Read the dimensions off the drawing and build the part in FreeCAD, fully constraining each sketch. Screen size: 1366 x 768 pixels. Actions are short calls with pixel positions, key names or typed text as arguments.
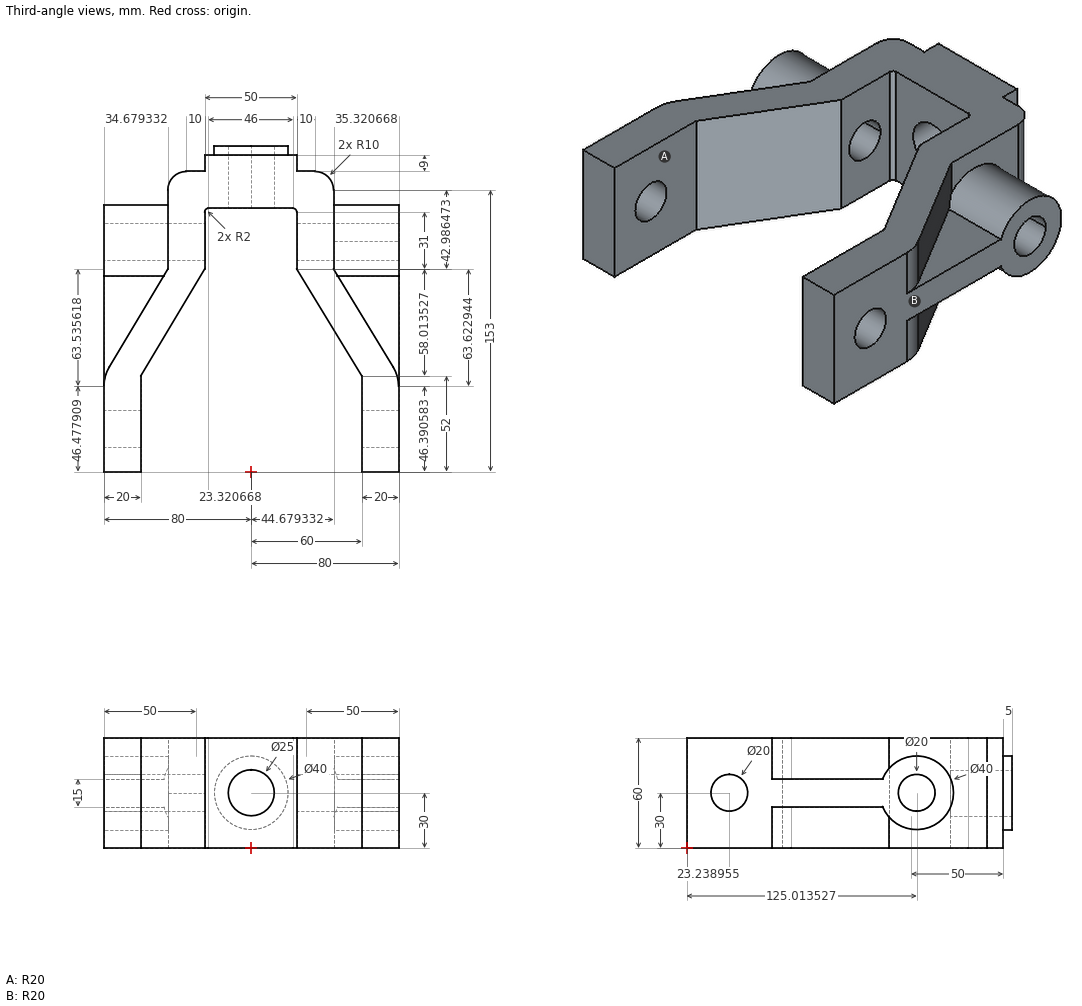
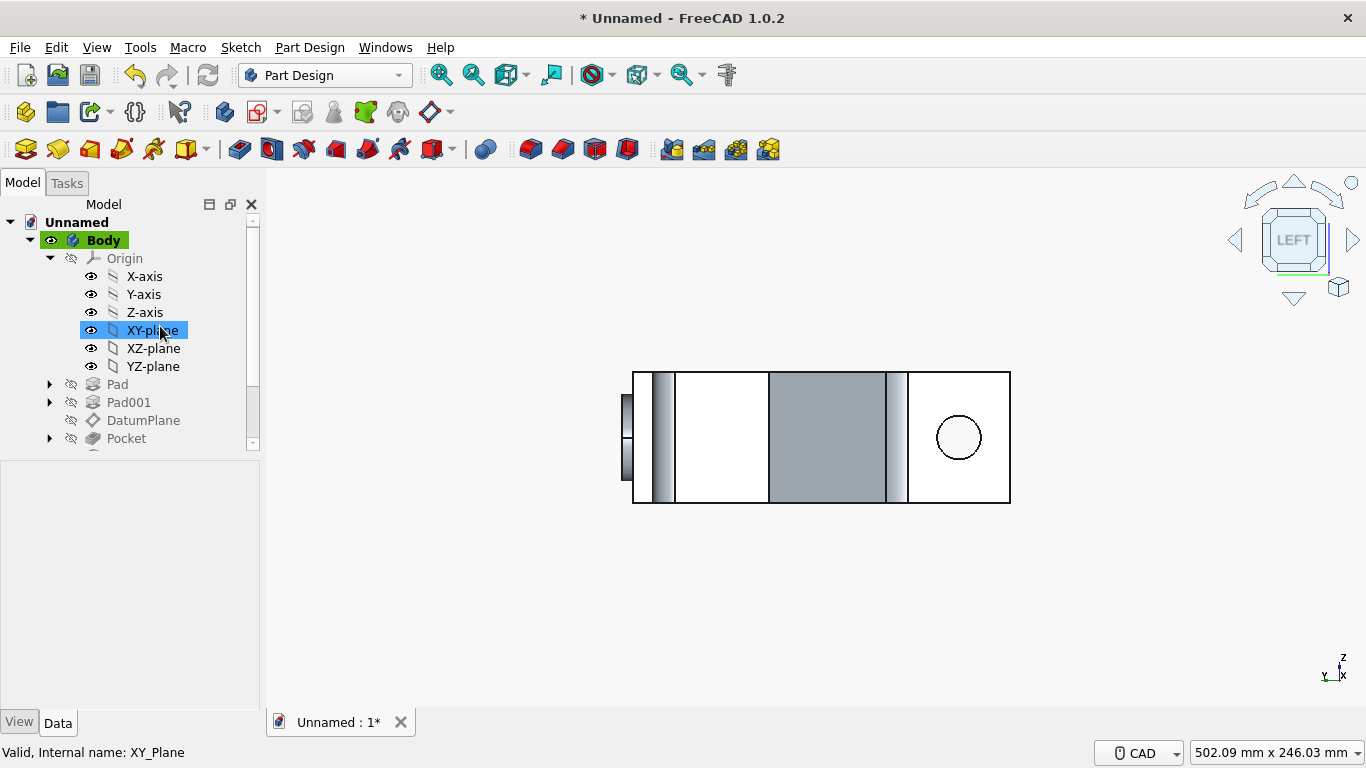
click(136, 366)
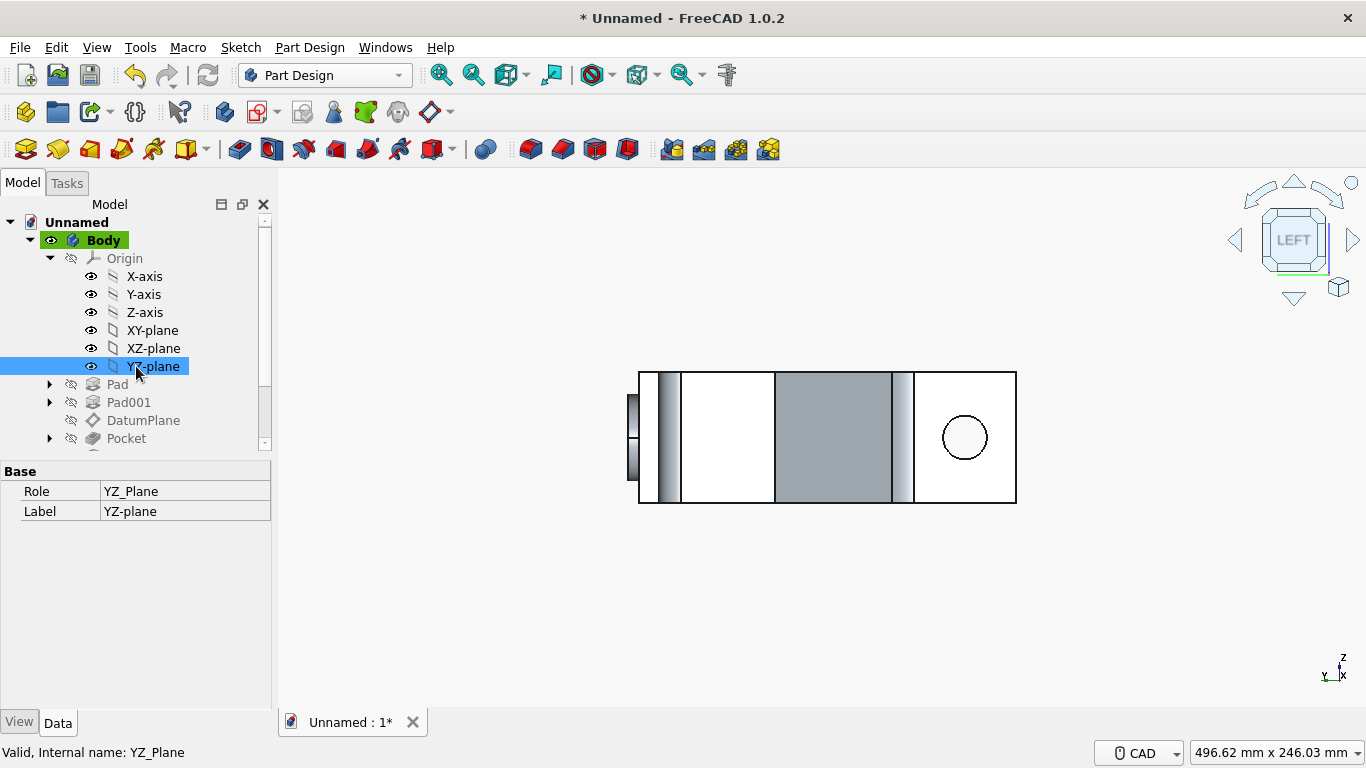
click(430, 112)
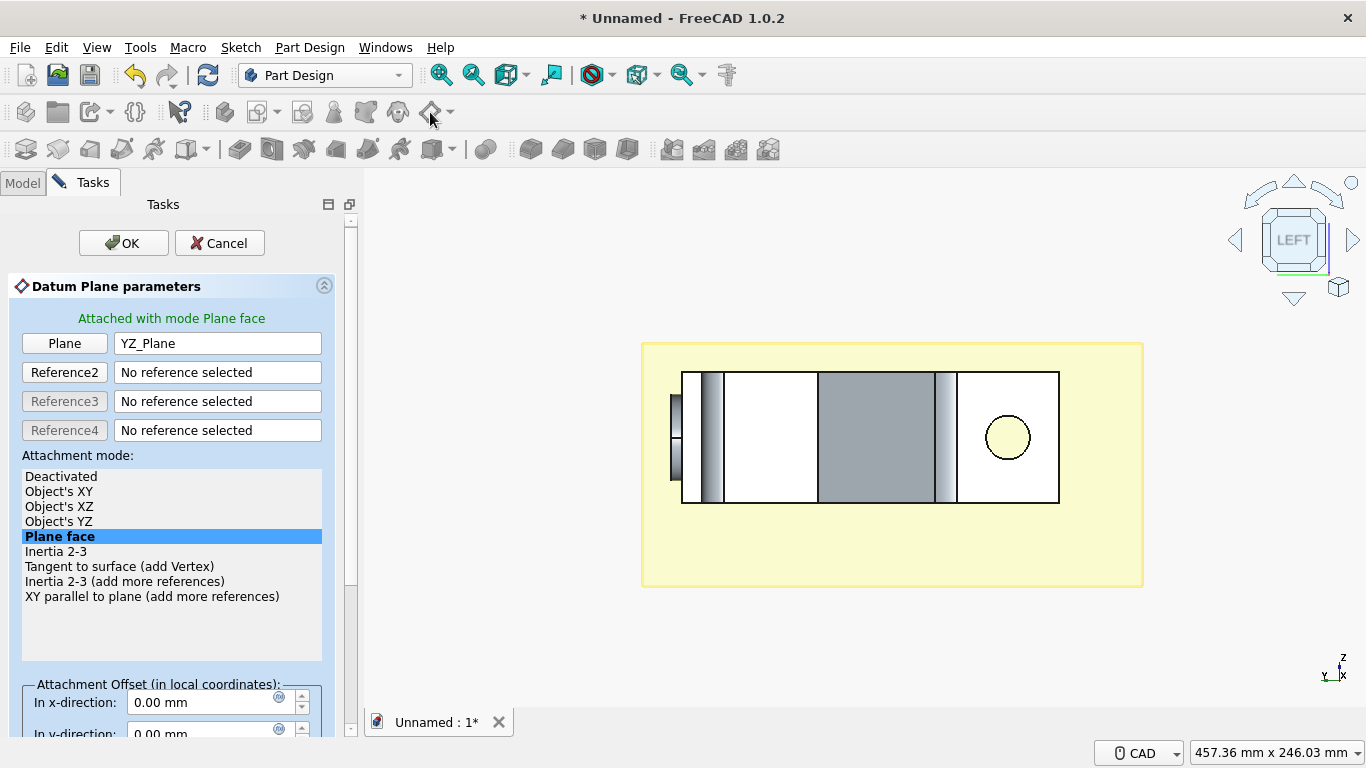
scroll(351, 475, down, 2)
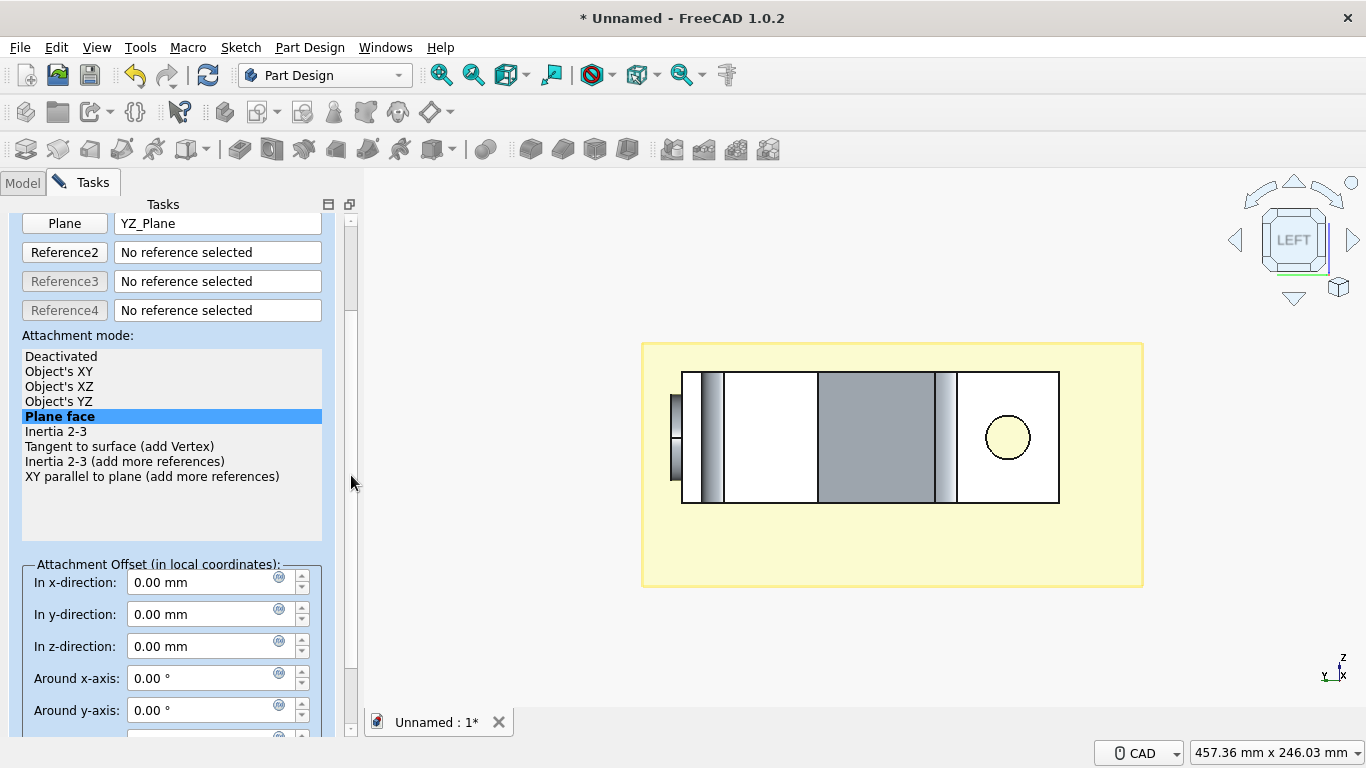
triple_click(210, 646)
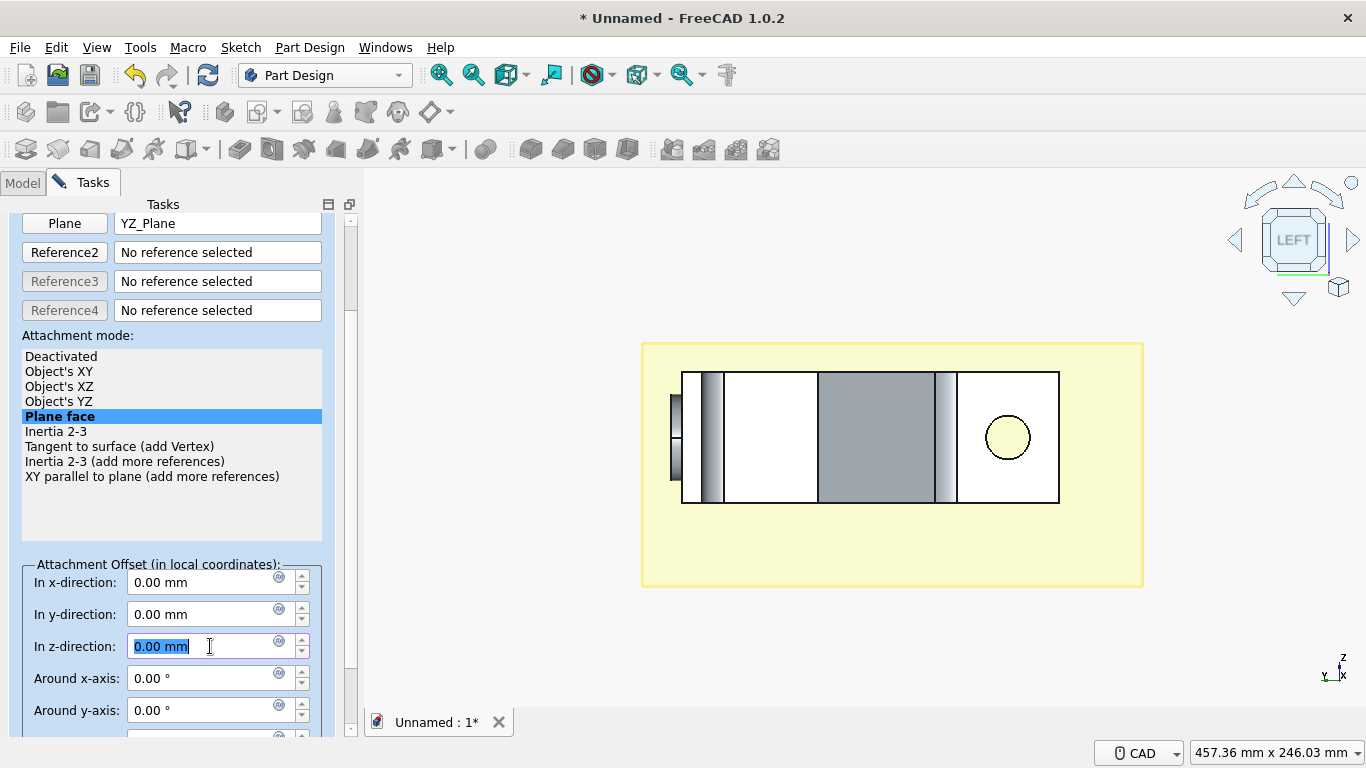
text(30)
key(Tab)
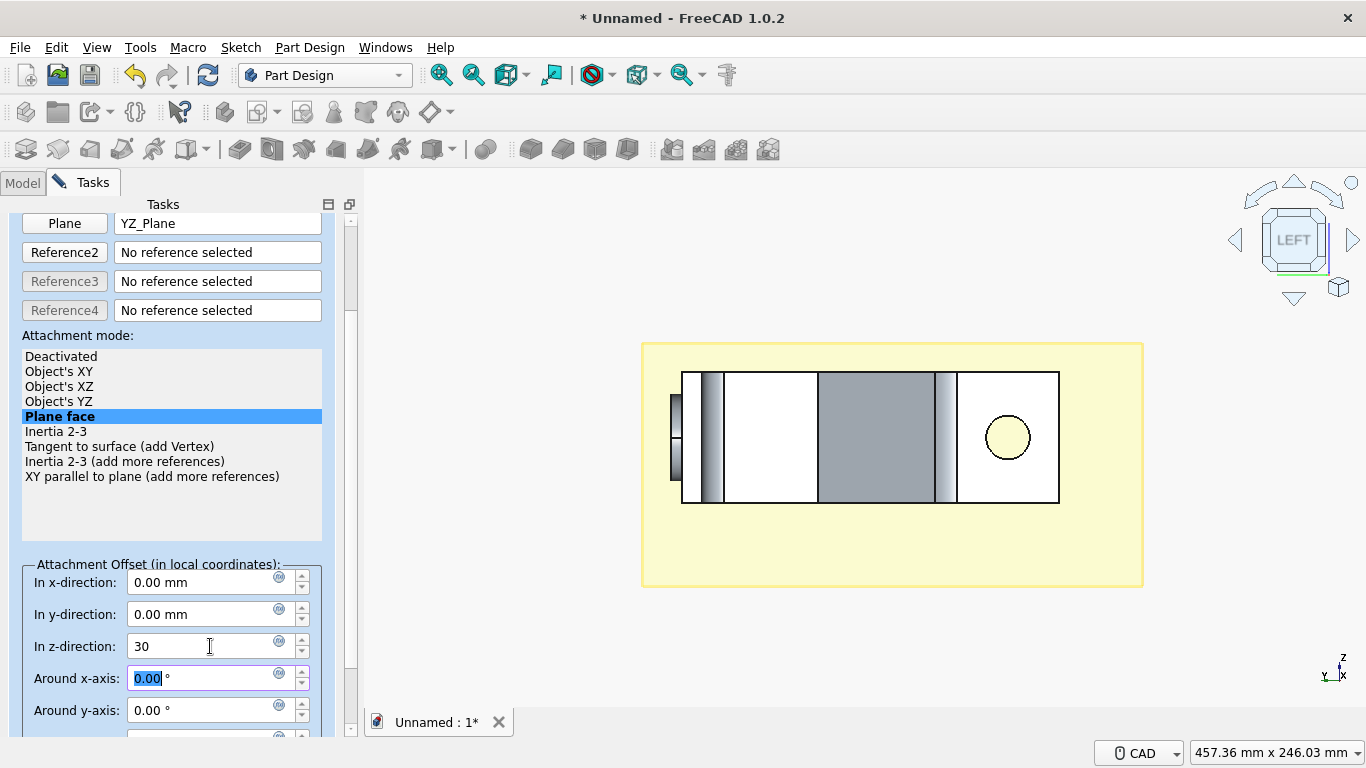
scroll(351, 475, up, 3)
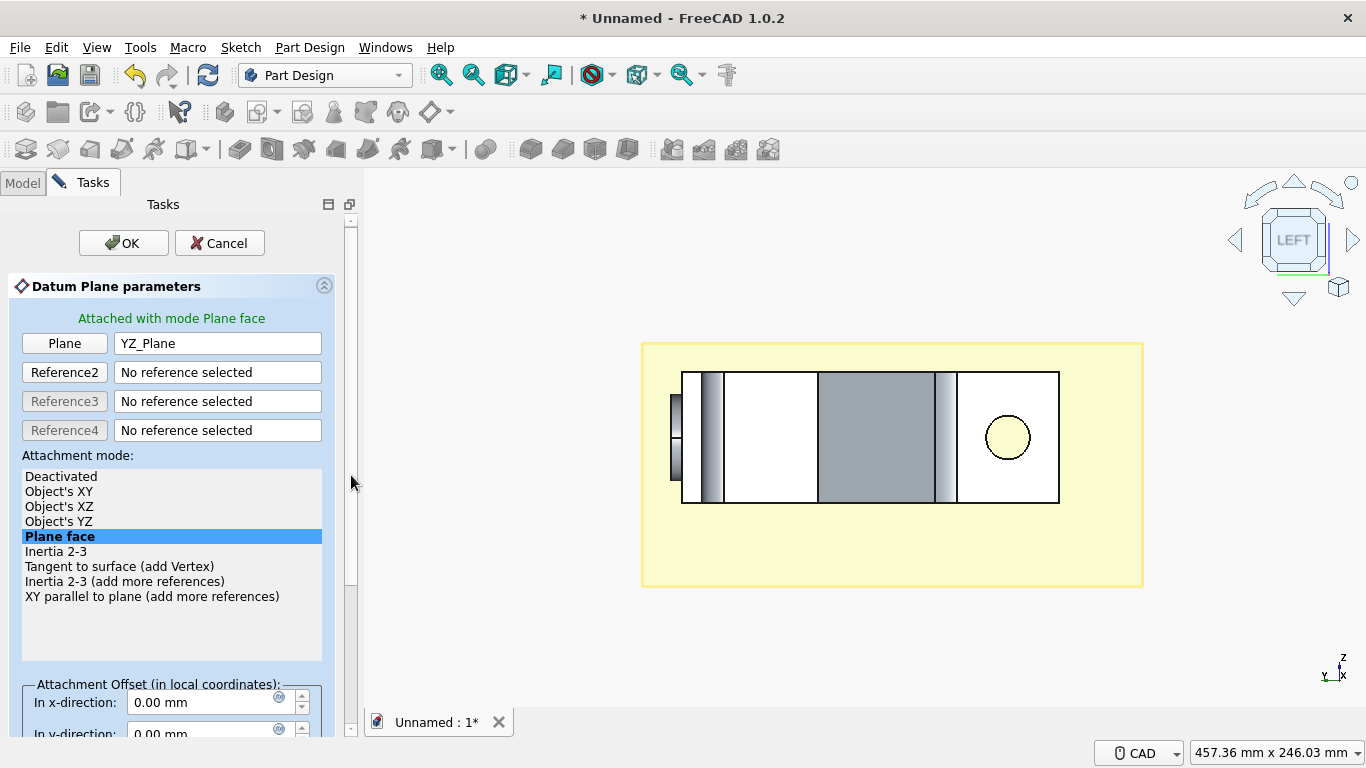
click(124, 243)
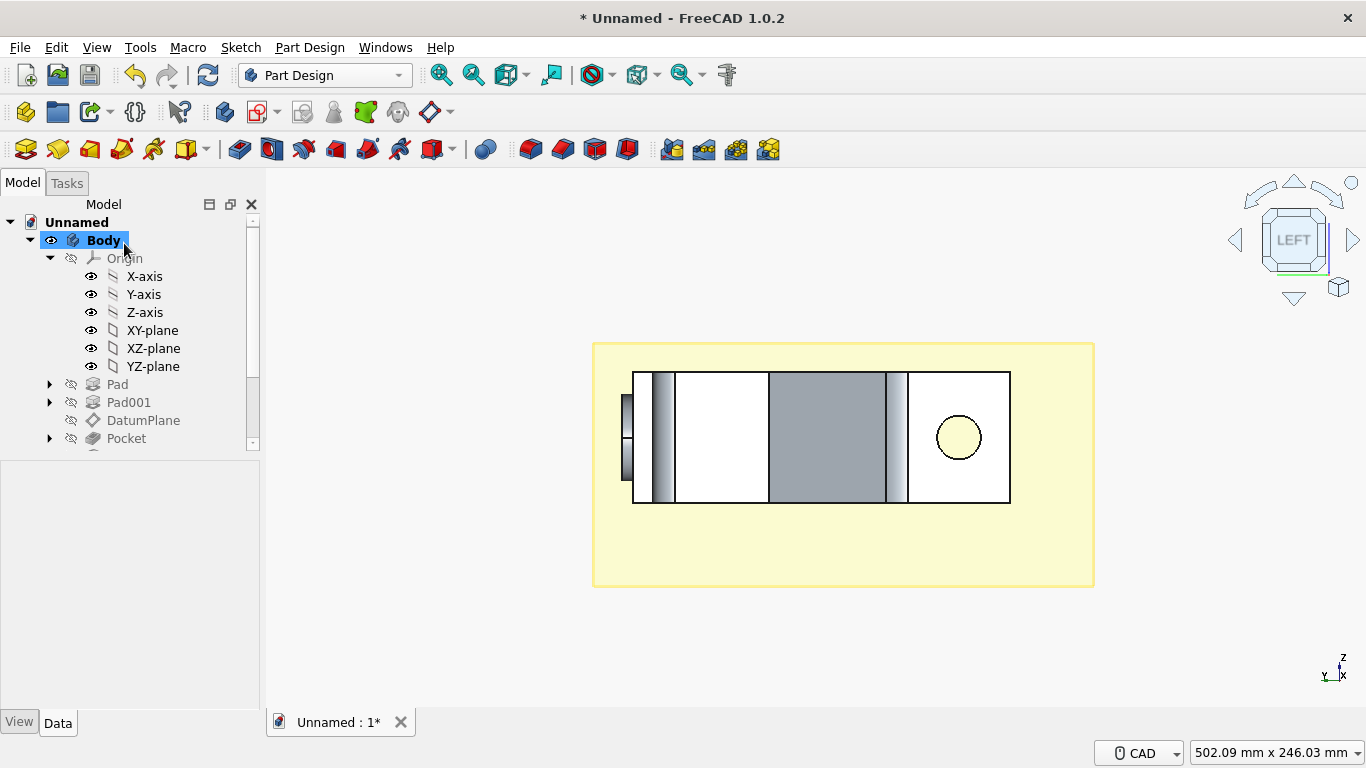
scroll(100, 326, down, 3)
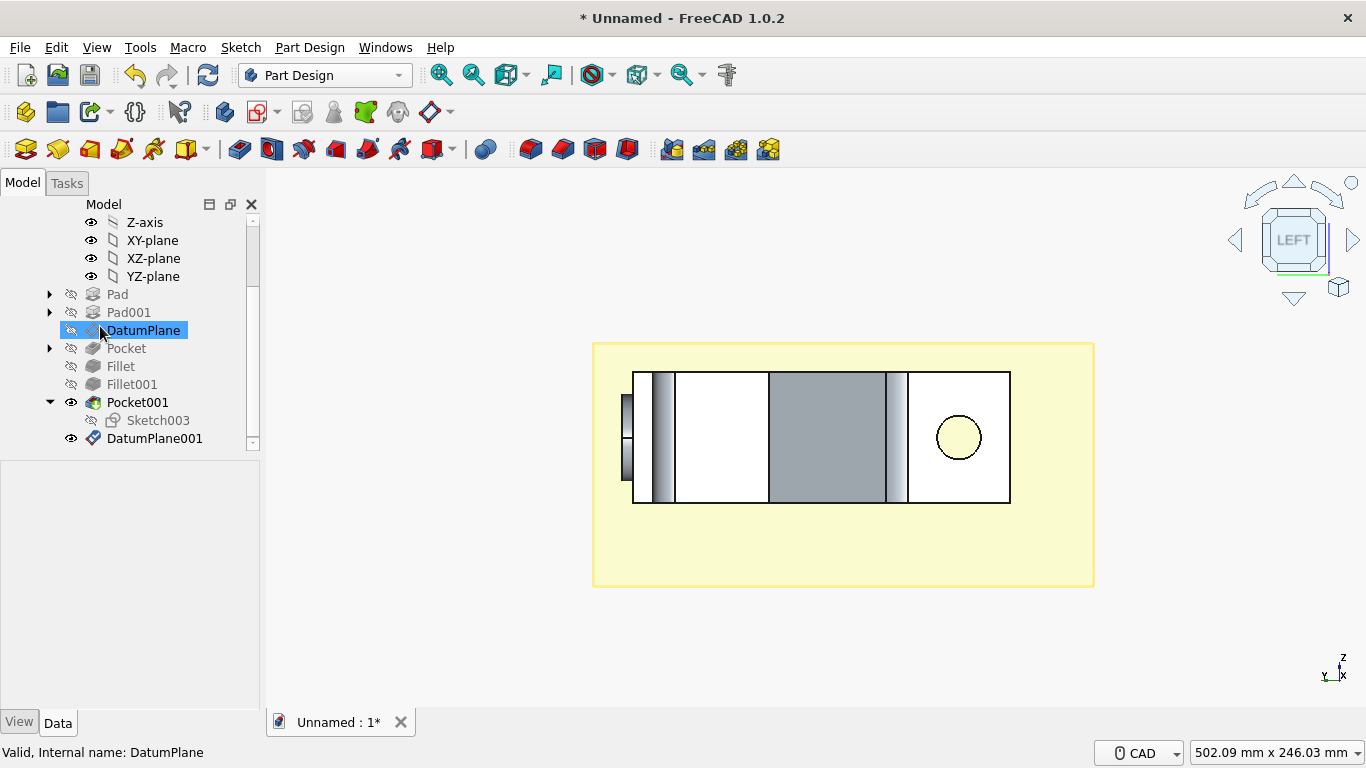
click(116, 438)